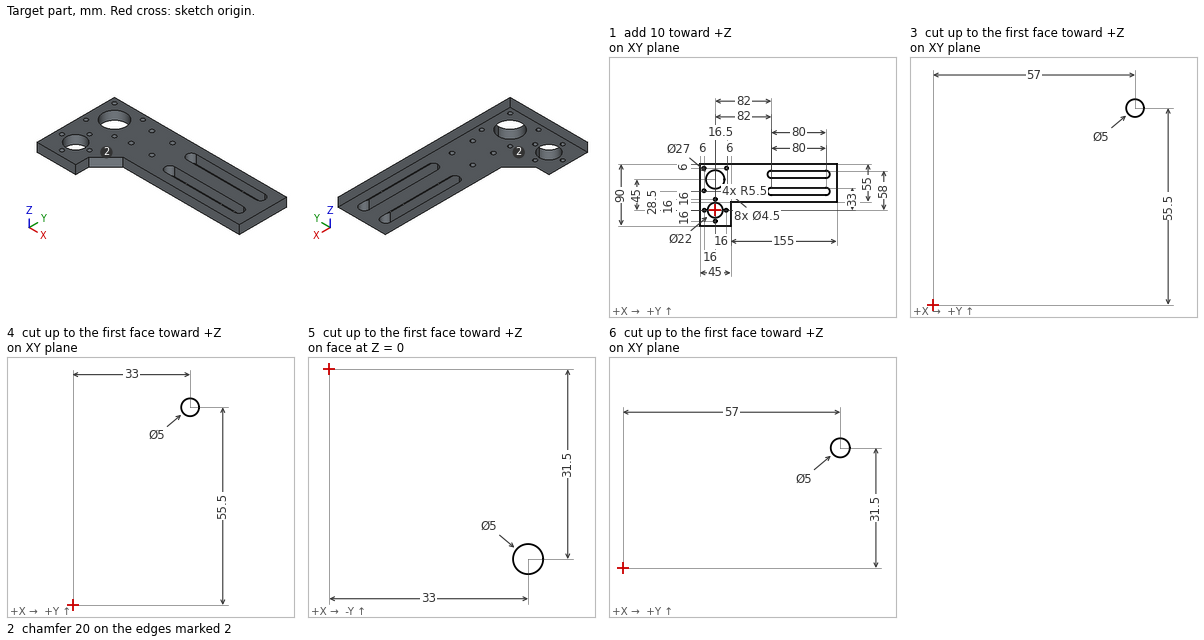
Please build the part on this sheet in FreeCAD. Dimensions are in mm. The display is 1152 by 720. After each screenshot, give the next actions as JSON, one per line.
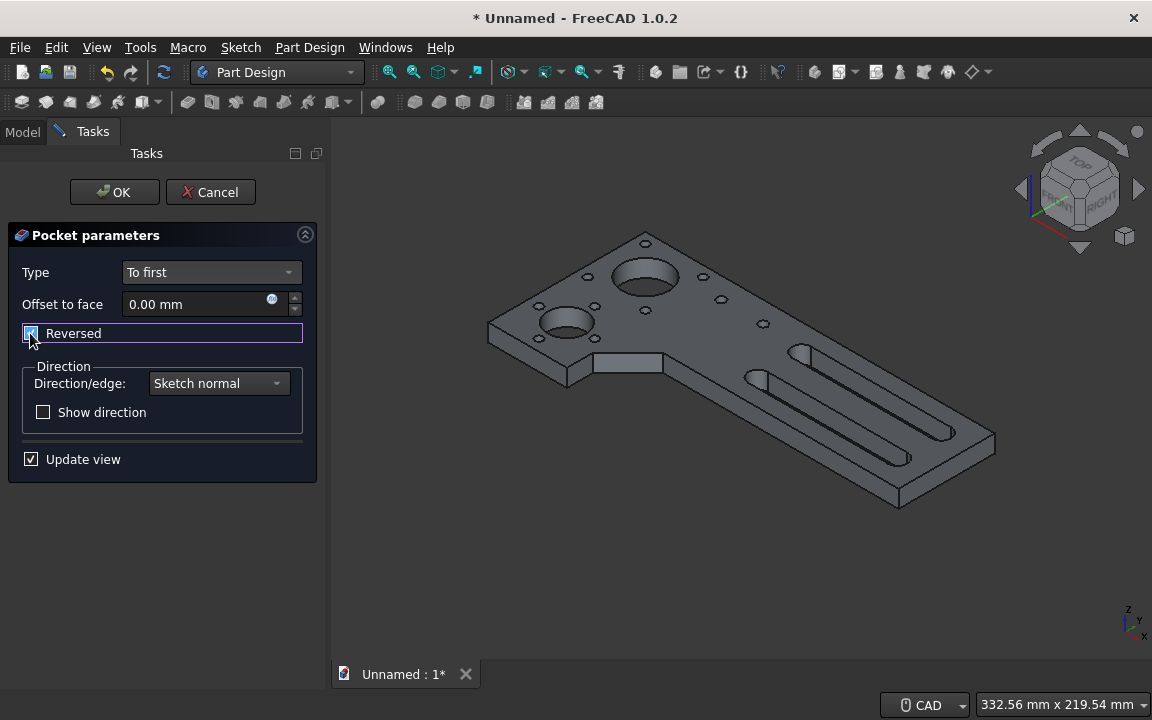
{"action": "left_click", "coordinate": [115, 192]}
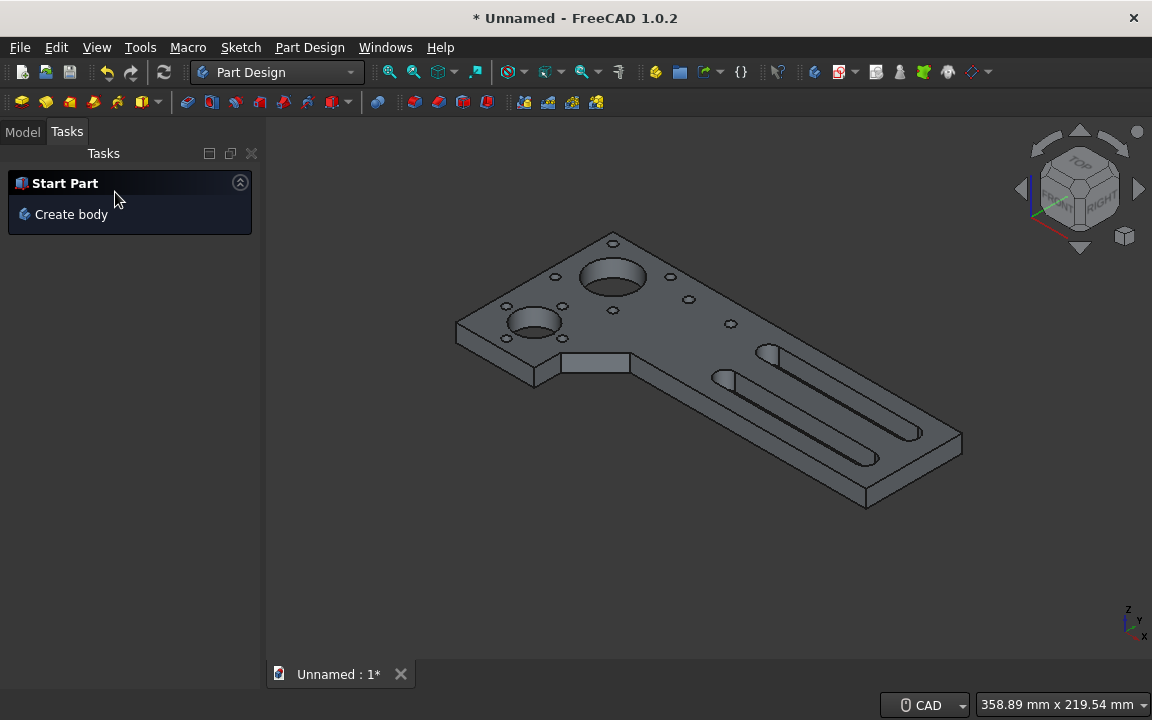
{"action": "key", "text": "5"}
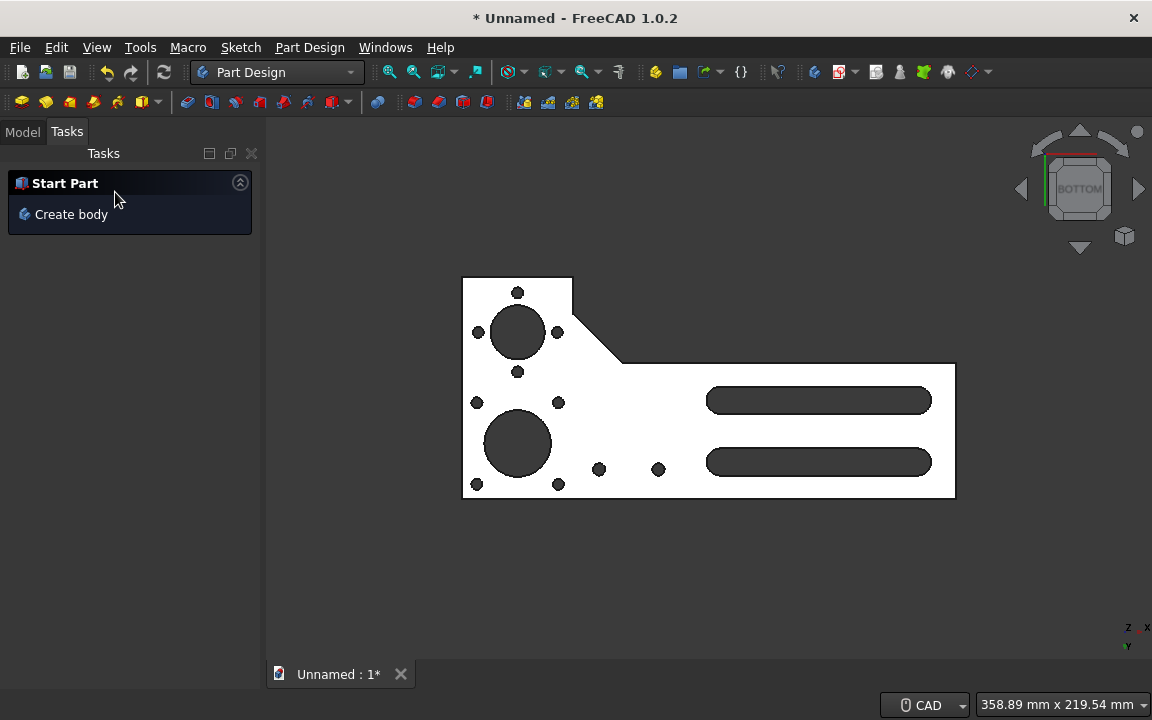
{"action": "left_click", "coordinate": [638, 419]}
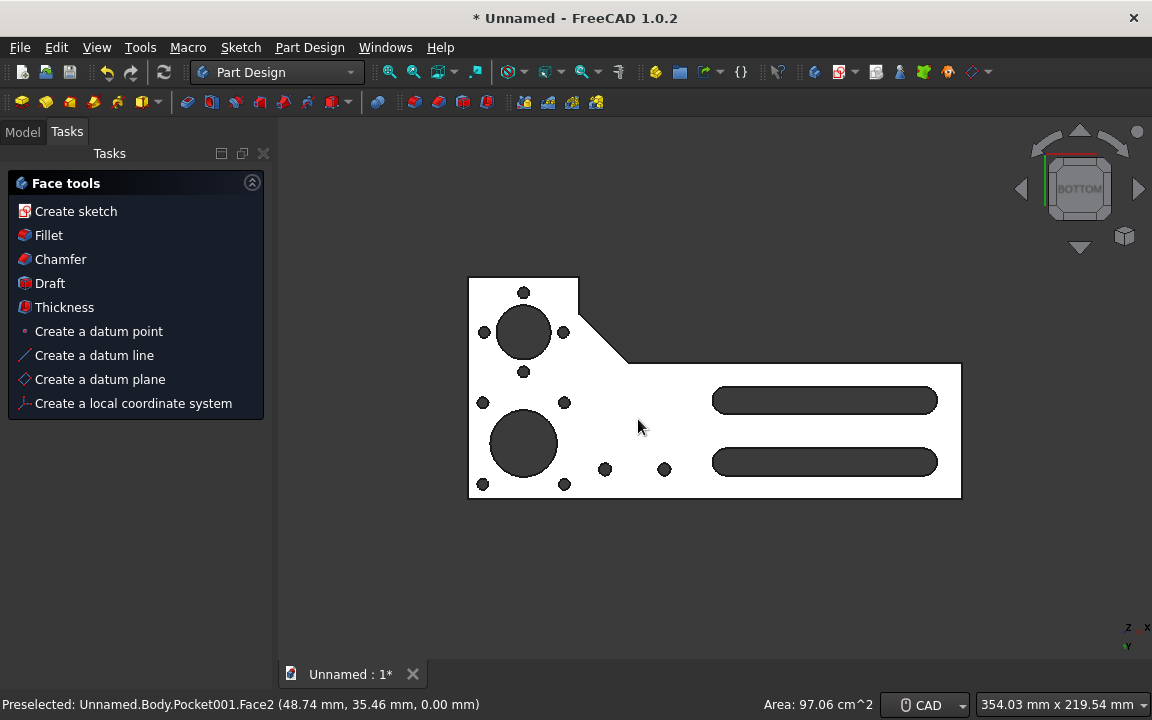
{"action": "left_click", "coordinate": [840, 72]}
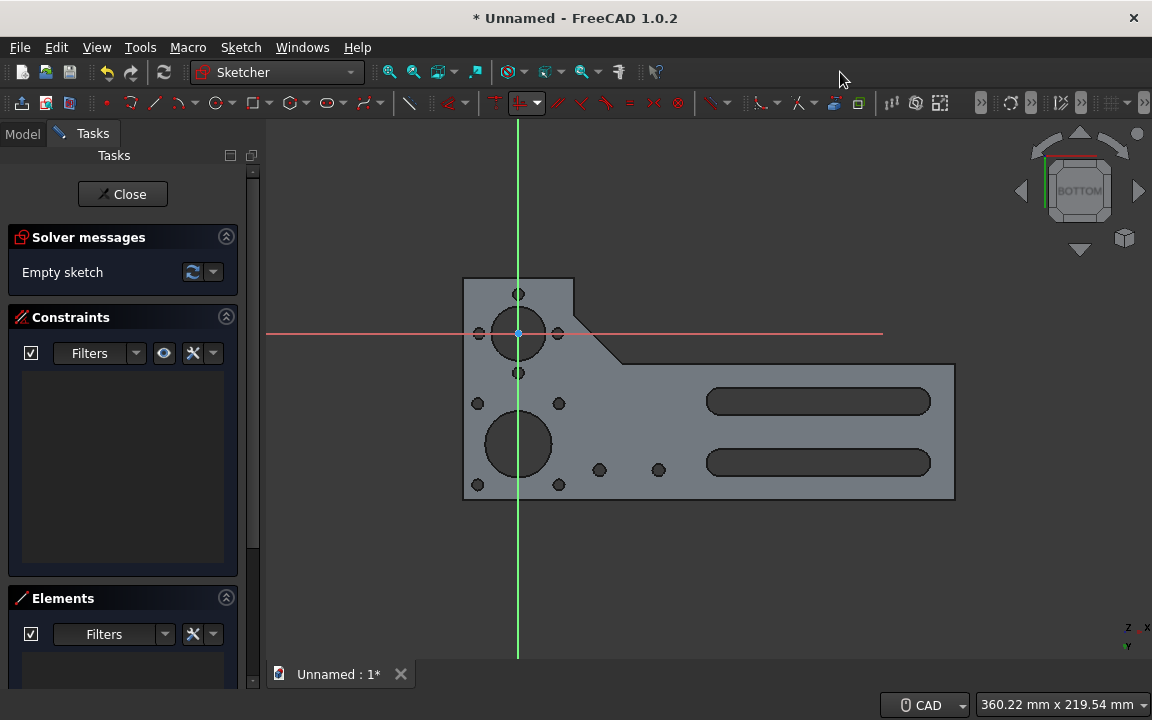
{"action": "scroll", "coordinate": [597, 412], "scroll_direction": "up", "scroll_amount": 15}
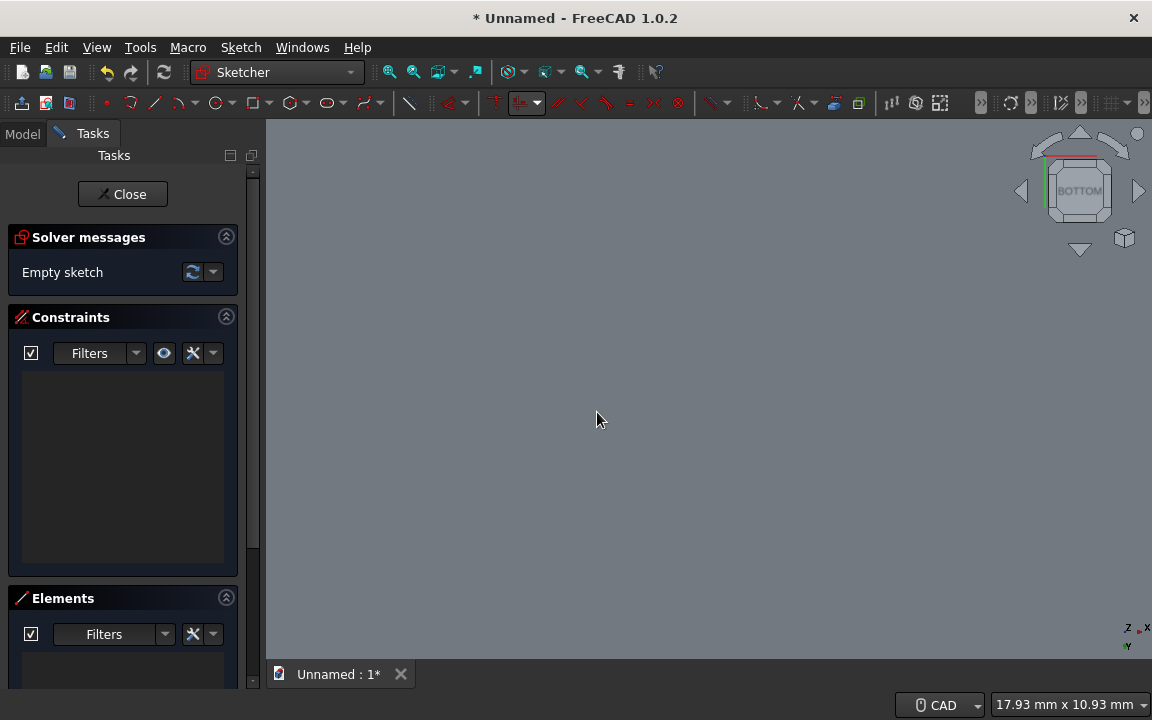
{"action": "scroll", "coordinate": [642, 375], "scroll_direction": "up", "scroll_amount": 2}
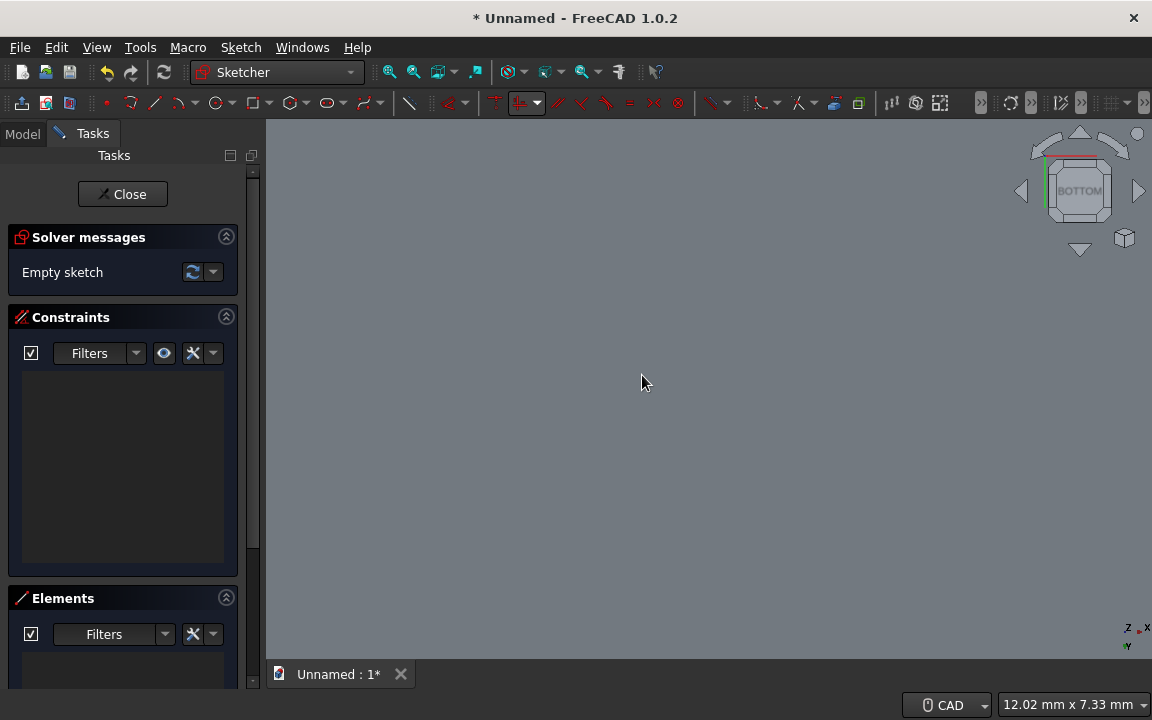
{"action": "key", "text": "g c"}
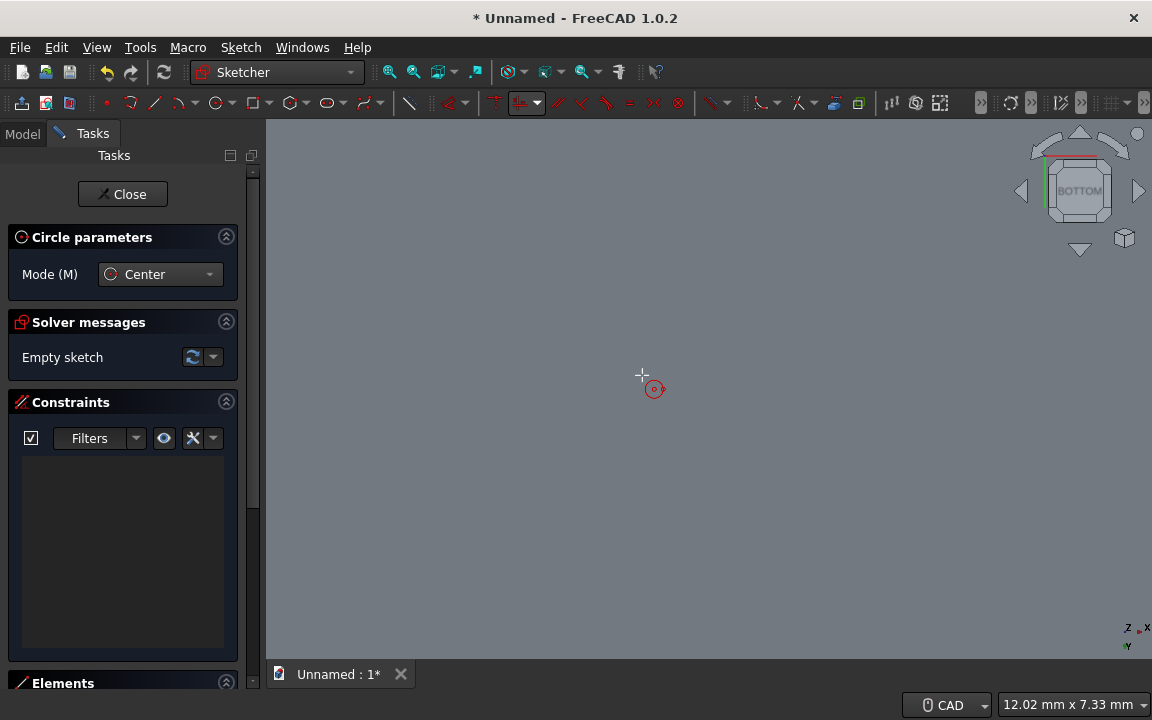
{"action": "left_click", "coordinate": [640, 389]}
{"action": "mouse_move", "coordinate": [771, 258]}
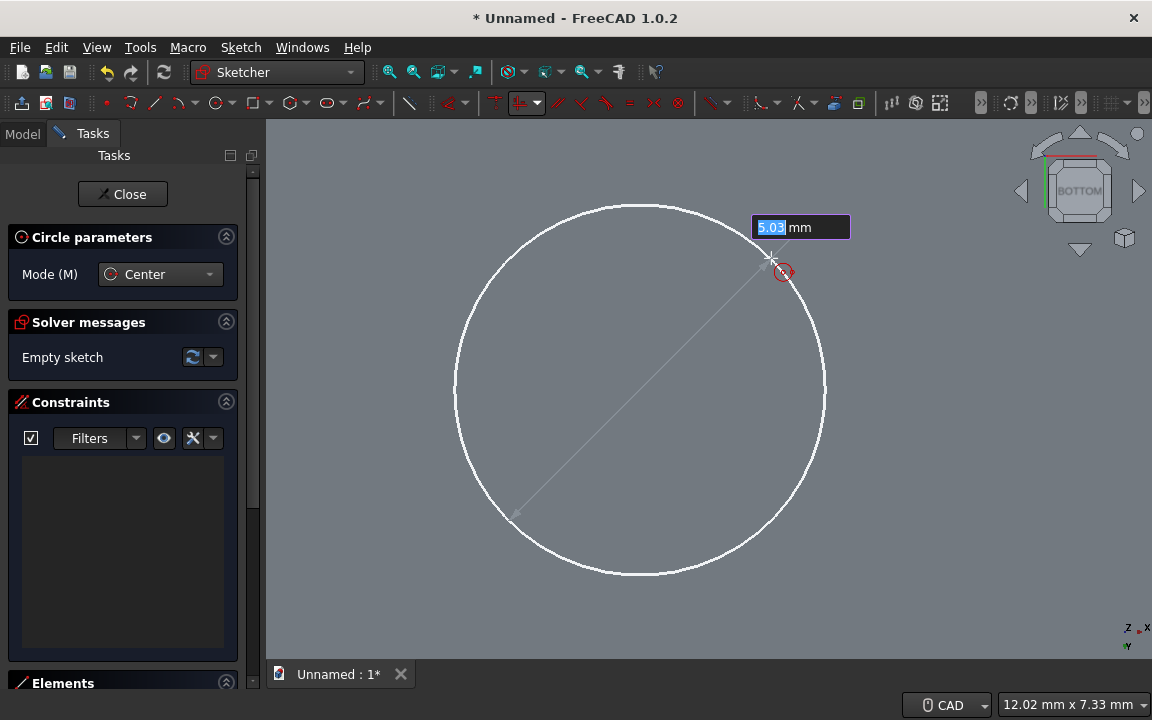
{"action": "type", "text": "5"}
{"action": "key", "text": "Return"}
{"action": "key", "text": "Escape"}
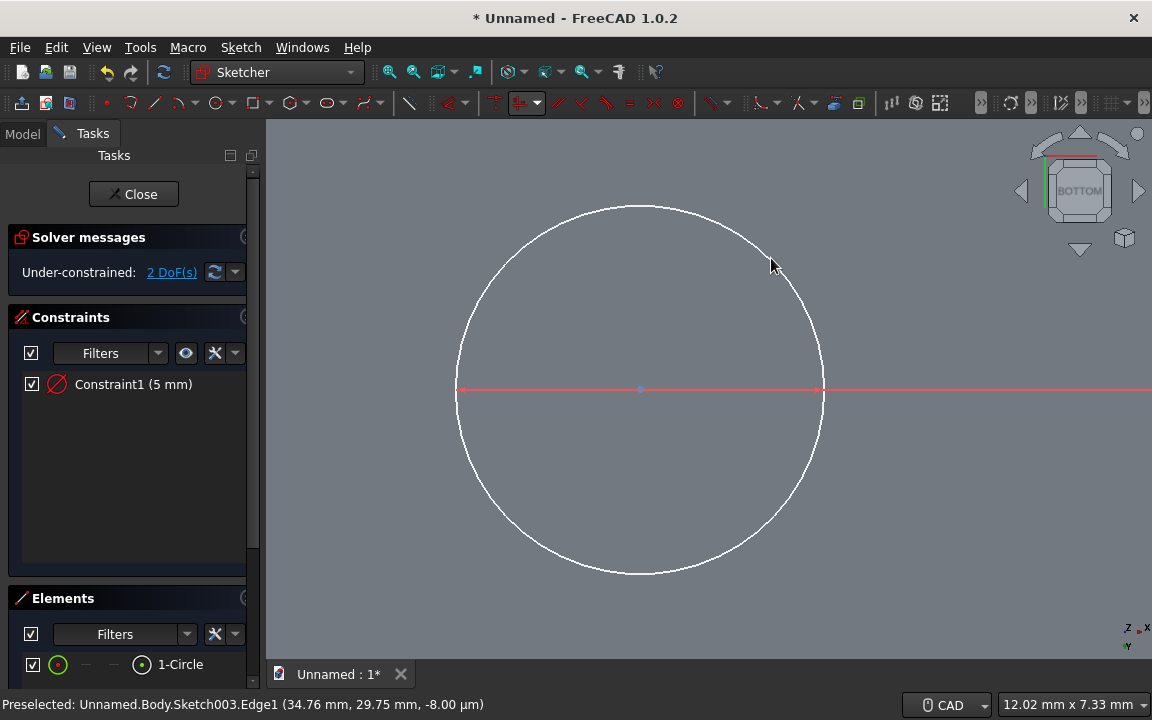
{"action": "key", "text": "d"}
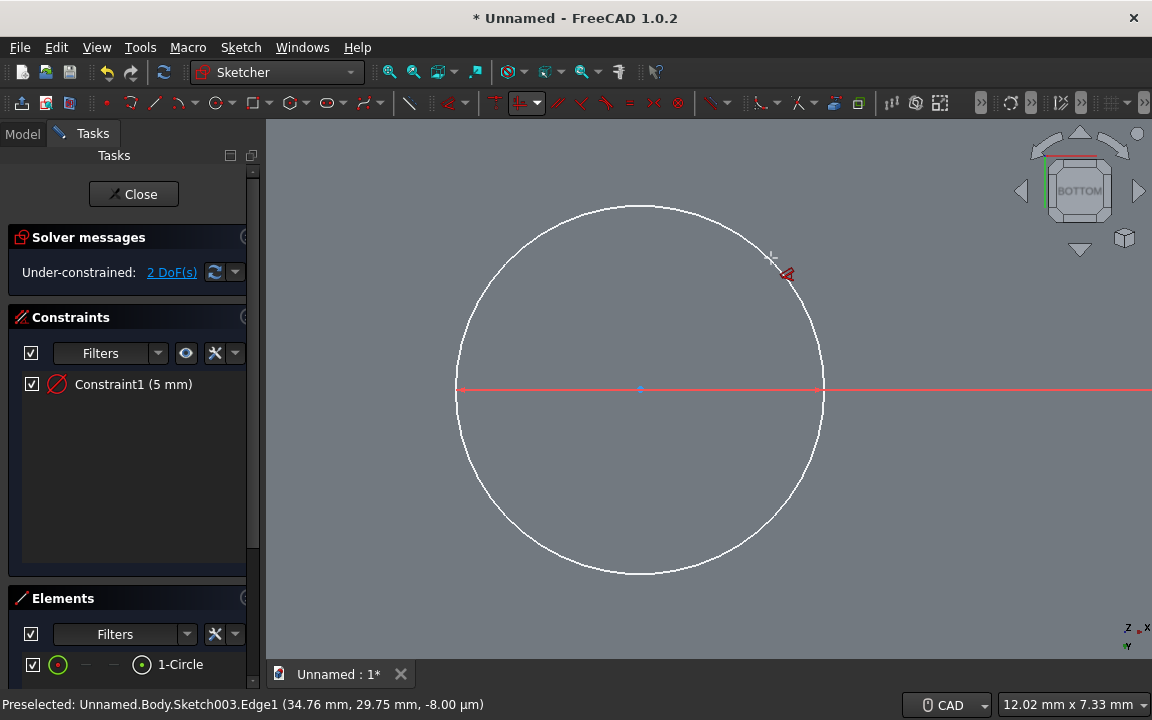
{"action": "left_click", "coordinate": [640, 390]}
{"action": "left_click", "coordinate": [387, 424]}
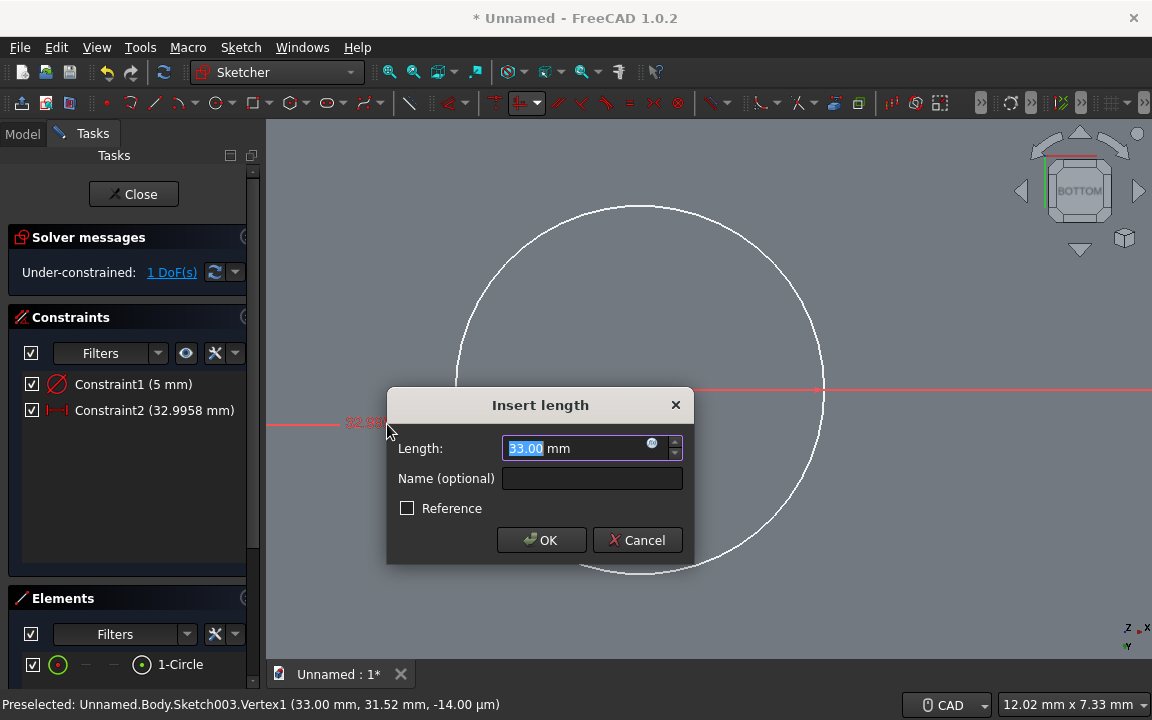
{"action": "type", "text": "33"}
{"action": "key", "text": "Return"}